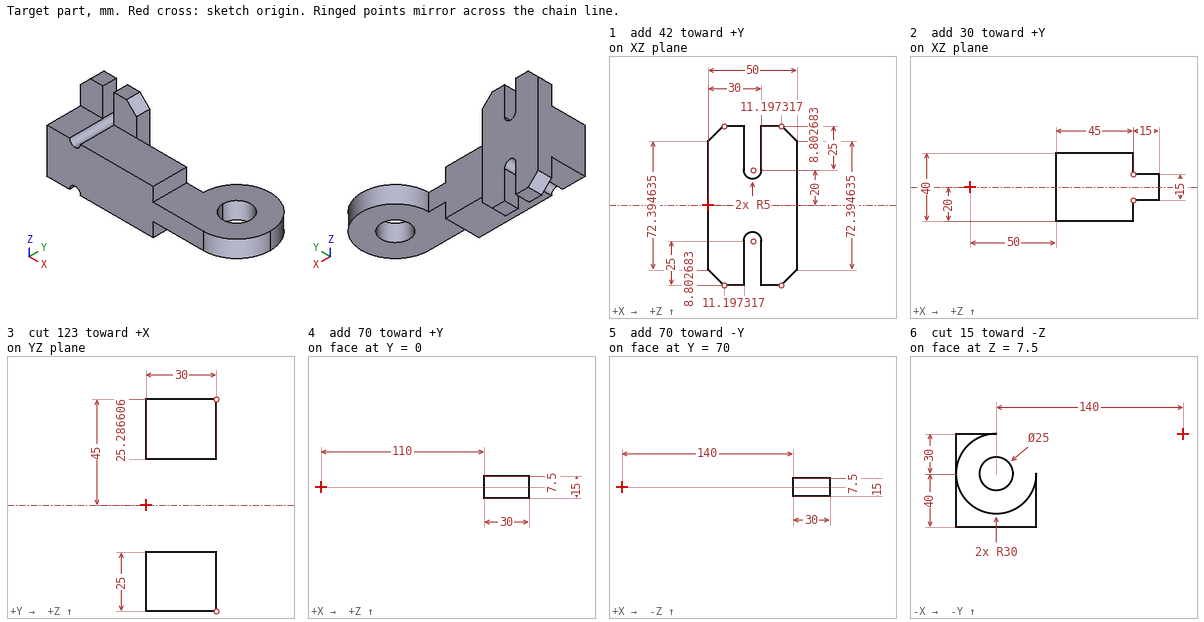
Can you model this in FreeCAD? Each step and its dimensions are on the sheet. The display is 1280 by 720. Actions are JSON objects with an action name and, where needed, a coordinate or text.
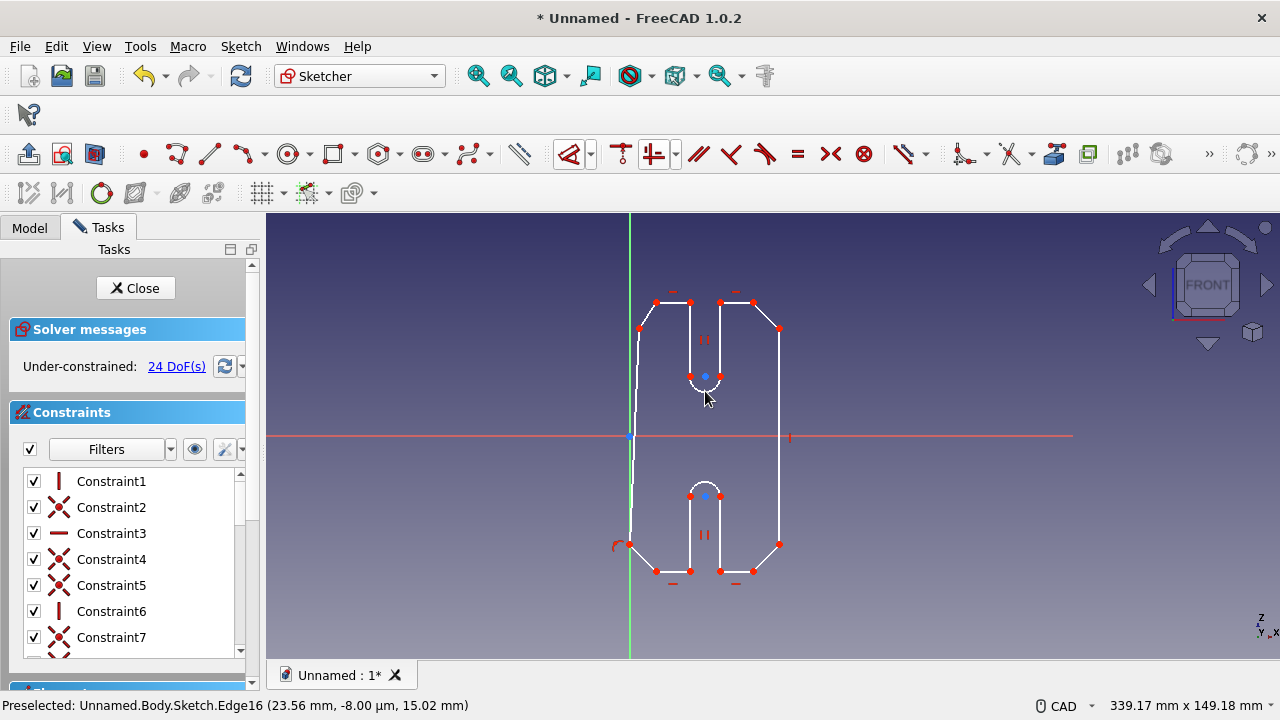
{"action": "left_click", "coordinate": [720, 355]}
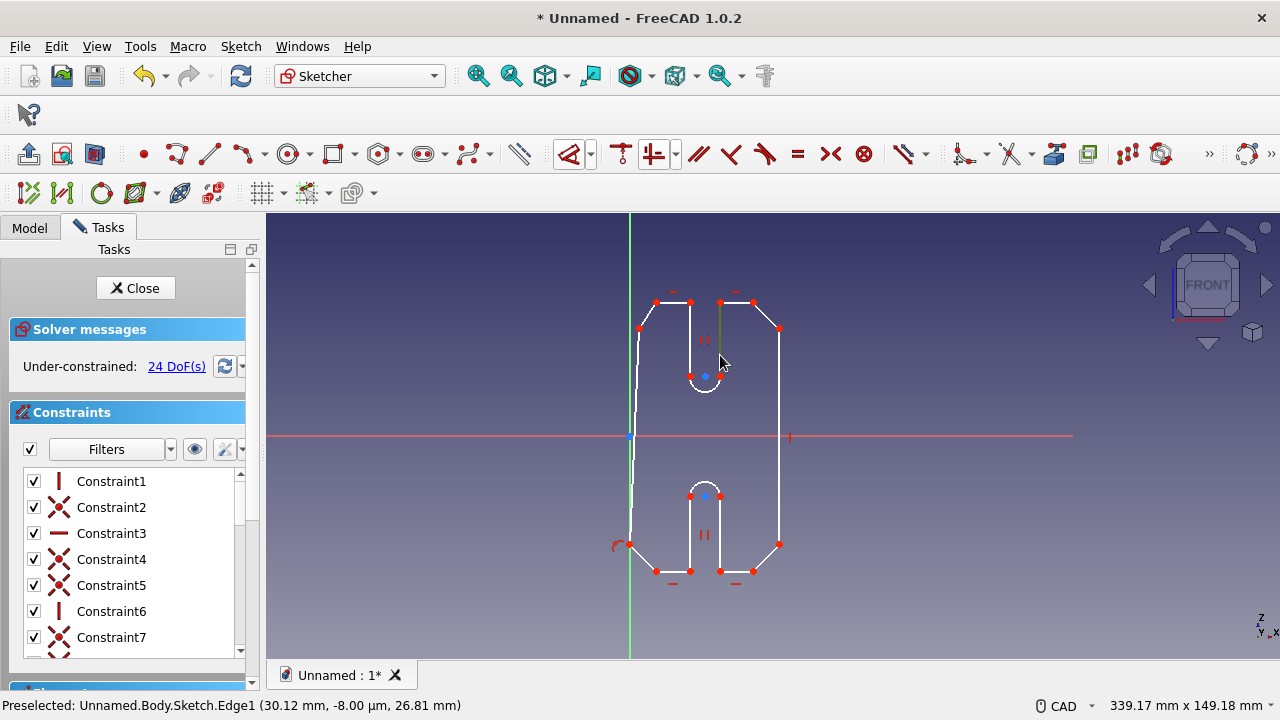
{"action": "left_click", "coordinate": [696, 389]}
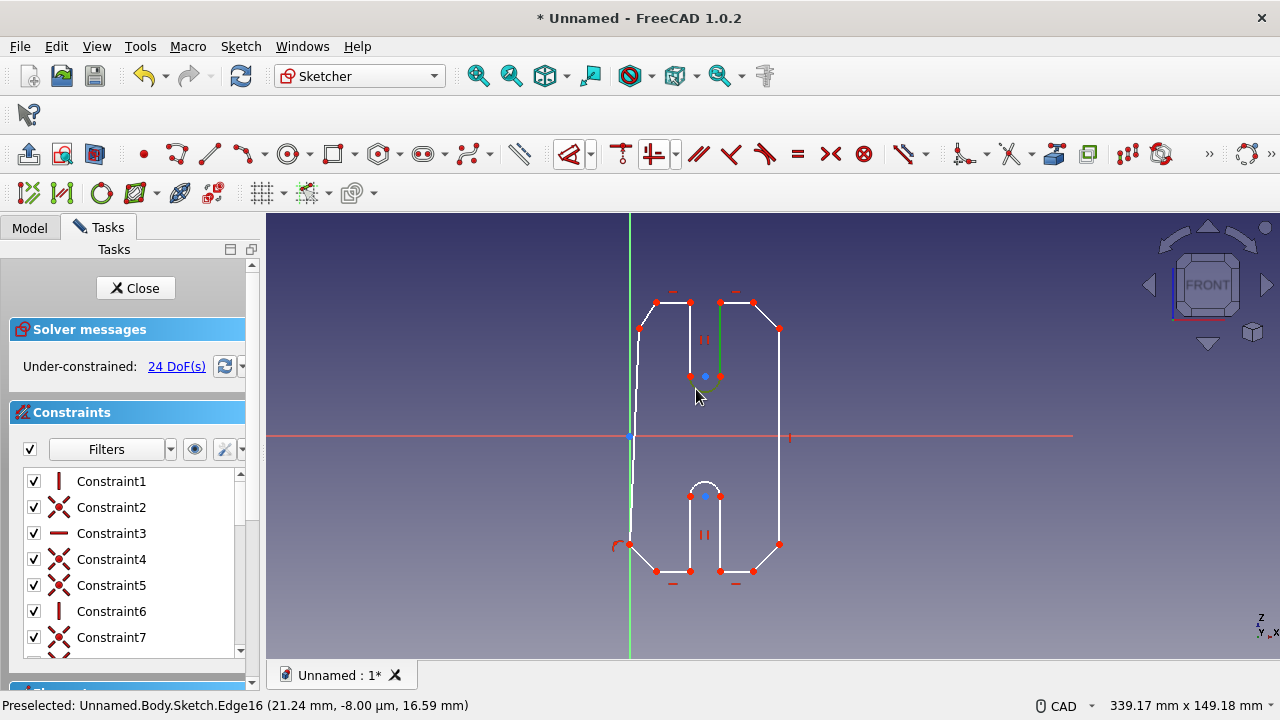
{"action": "left_click", "coordinate": [765, 154]}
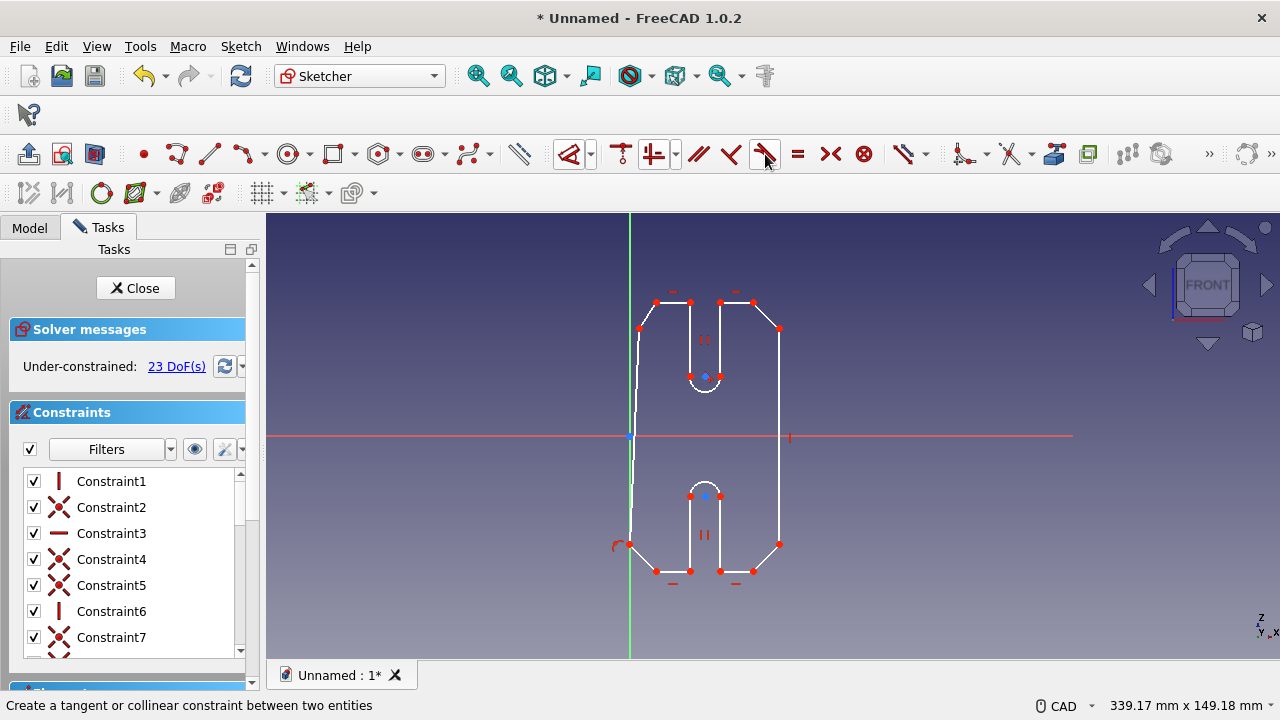
{"action": "left_click", "coordinate": [720, 549]}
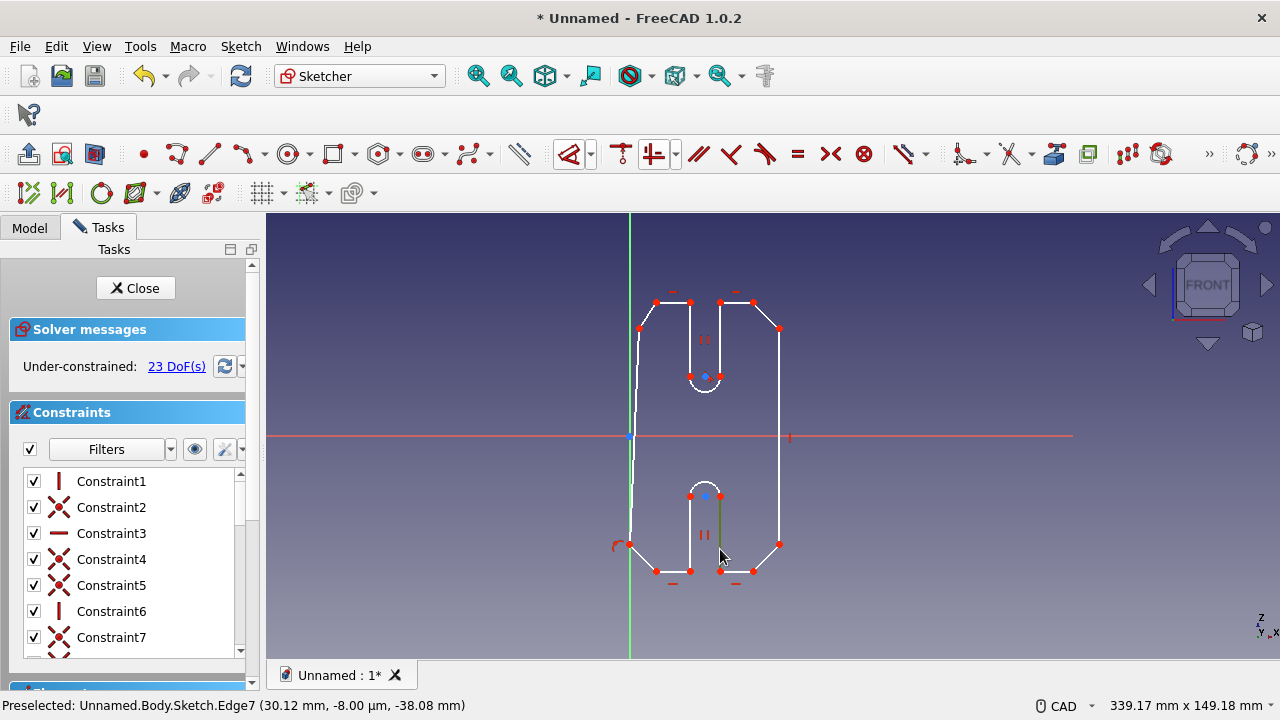
{"action": "left_click", "coordinate": [714, 485]}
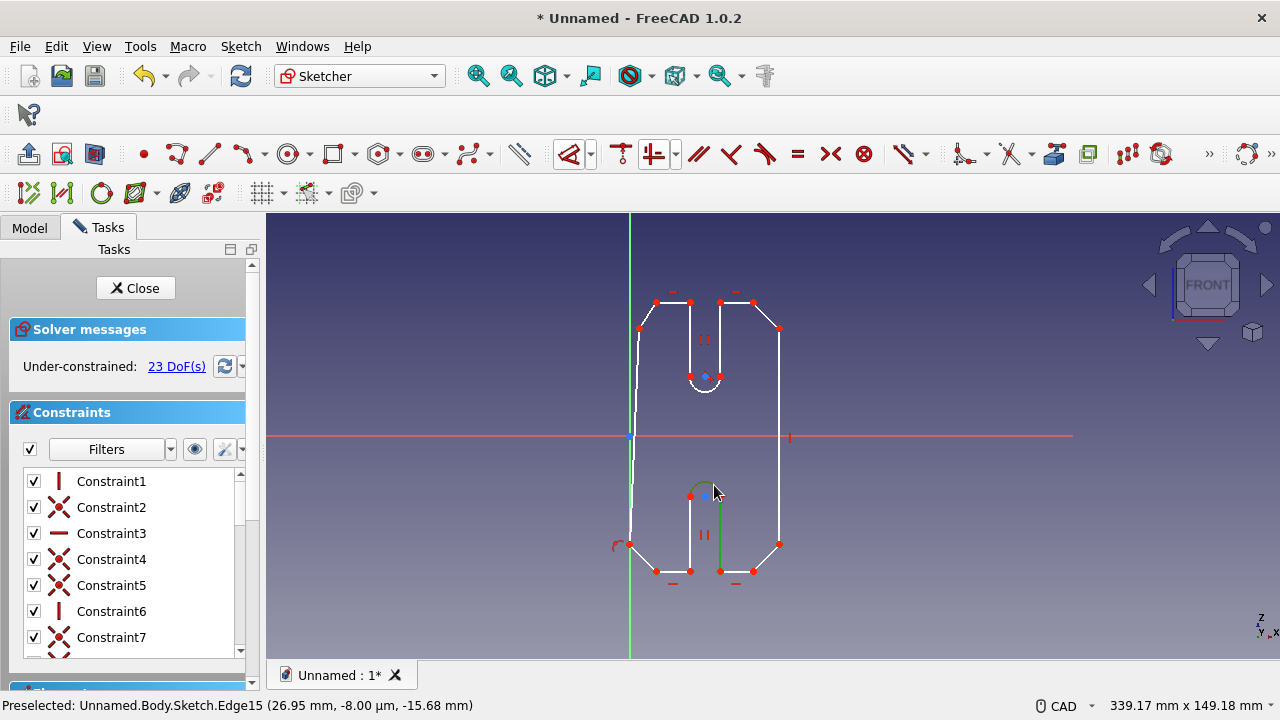
{"action": "key", "text": "t"}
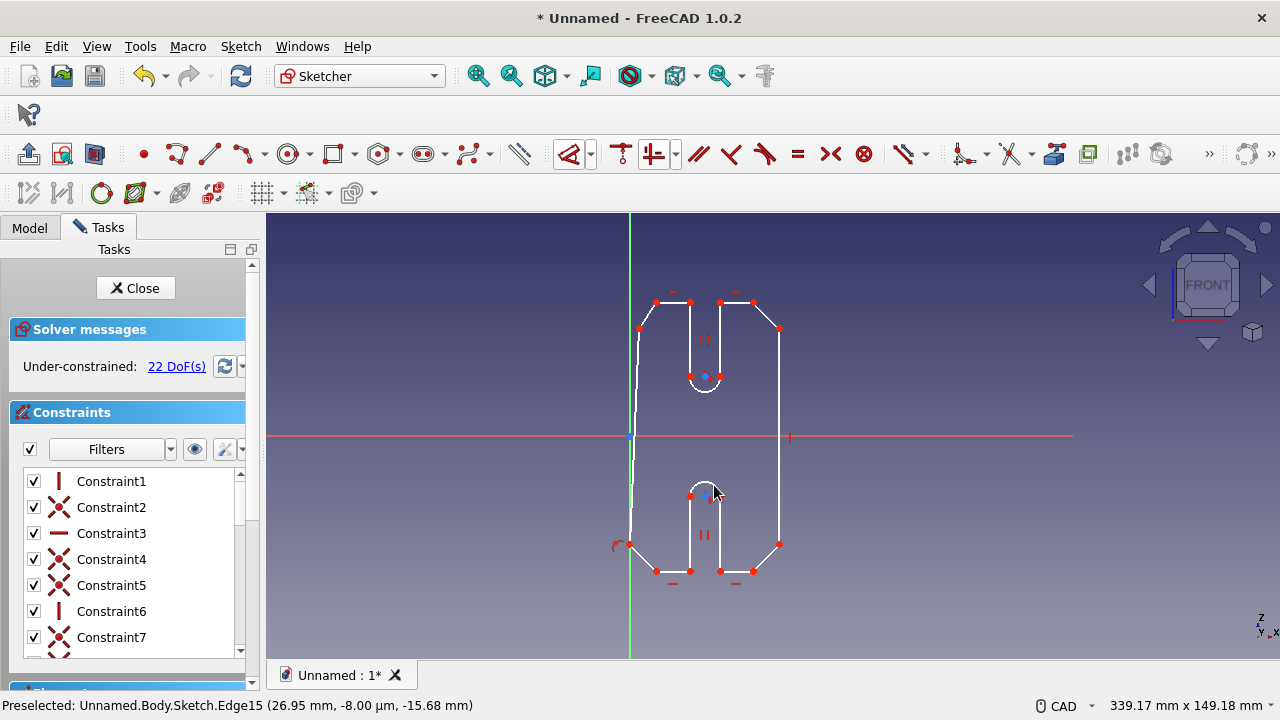
{"action": "left_click", "coordinate": [690, 519]}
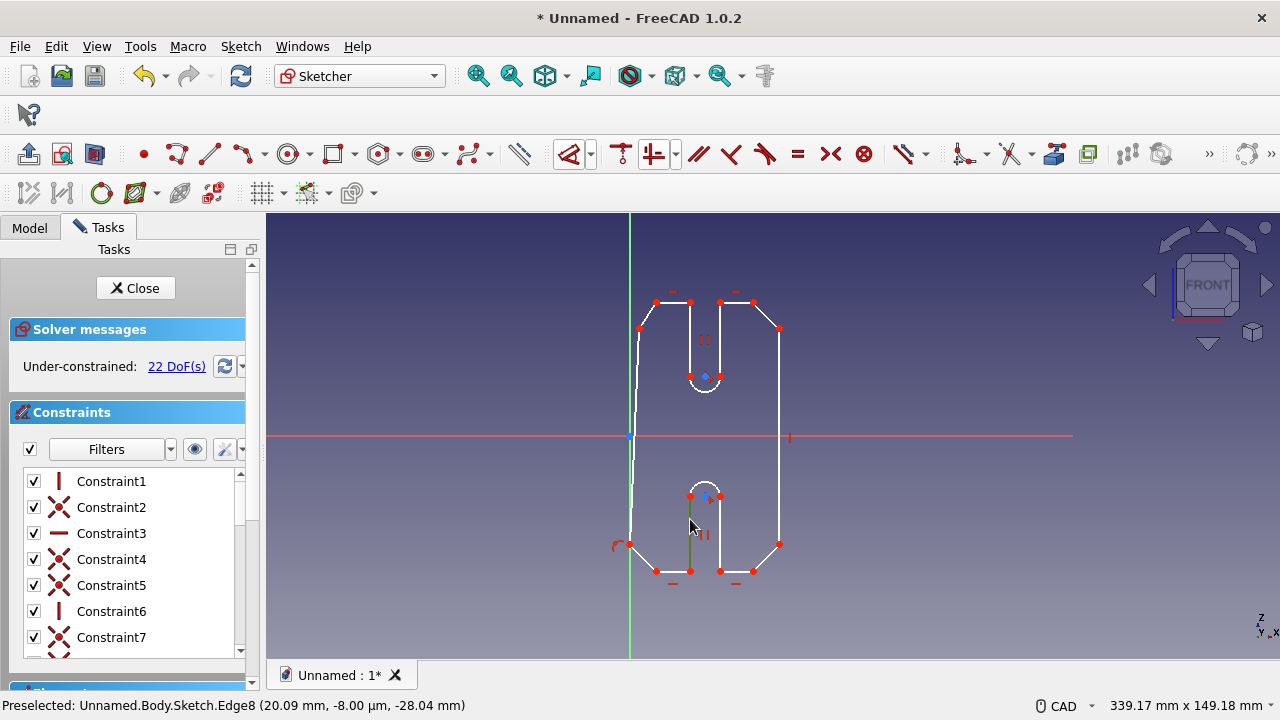
{"action": "left_click", "coordinate": [714, 485]}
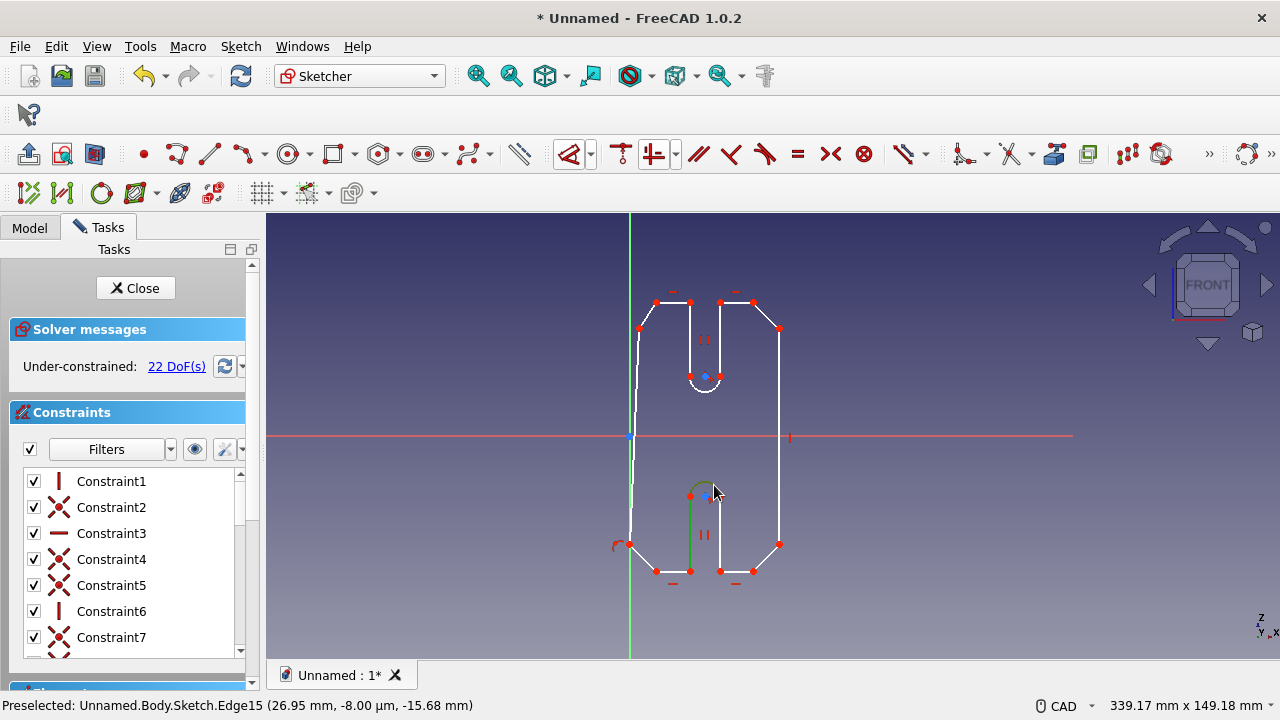
{"action": "left_click", "coordinate": [765, 154]}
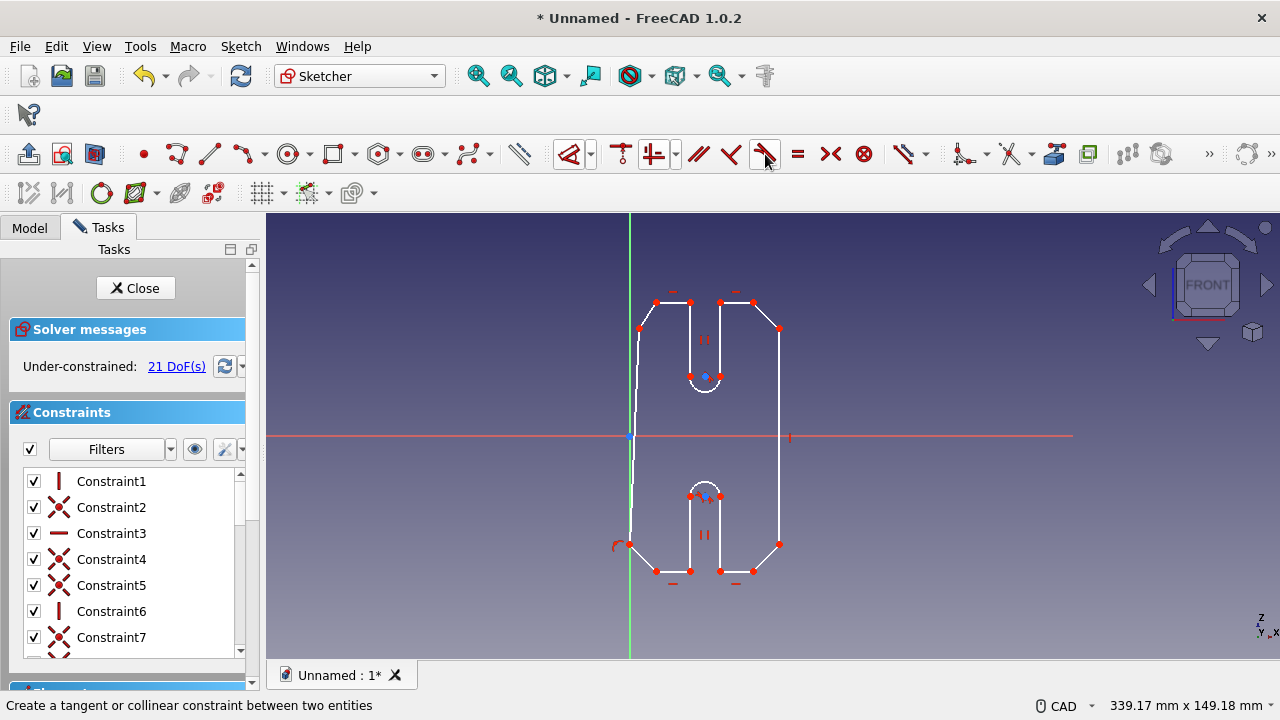
{"action": "left_click", "coordinate": [690, 325]}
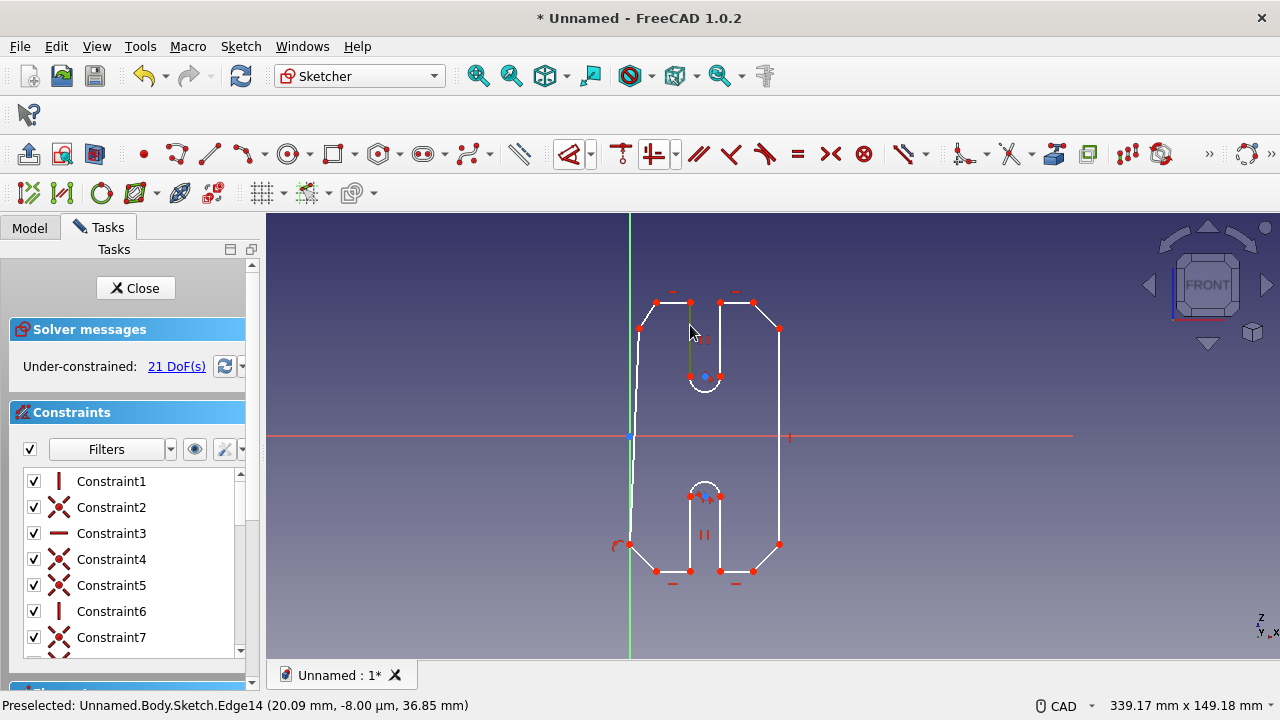
{"action": "left_click", "coordinate": [696, 389]}